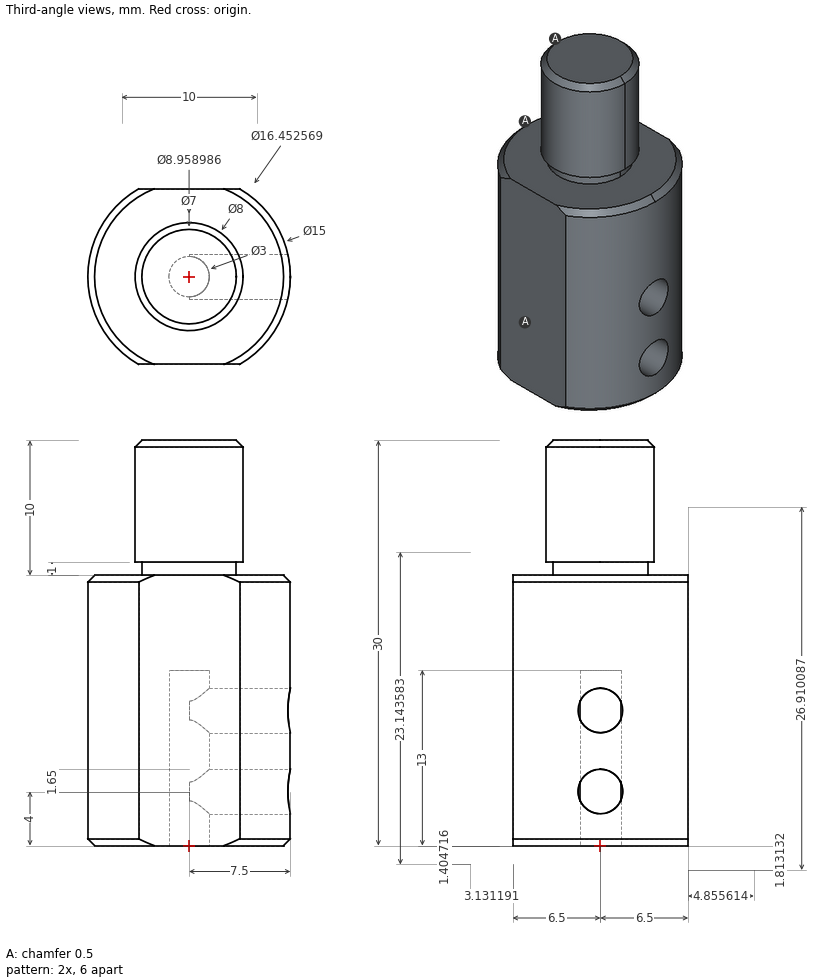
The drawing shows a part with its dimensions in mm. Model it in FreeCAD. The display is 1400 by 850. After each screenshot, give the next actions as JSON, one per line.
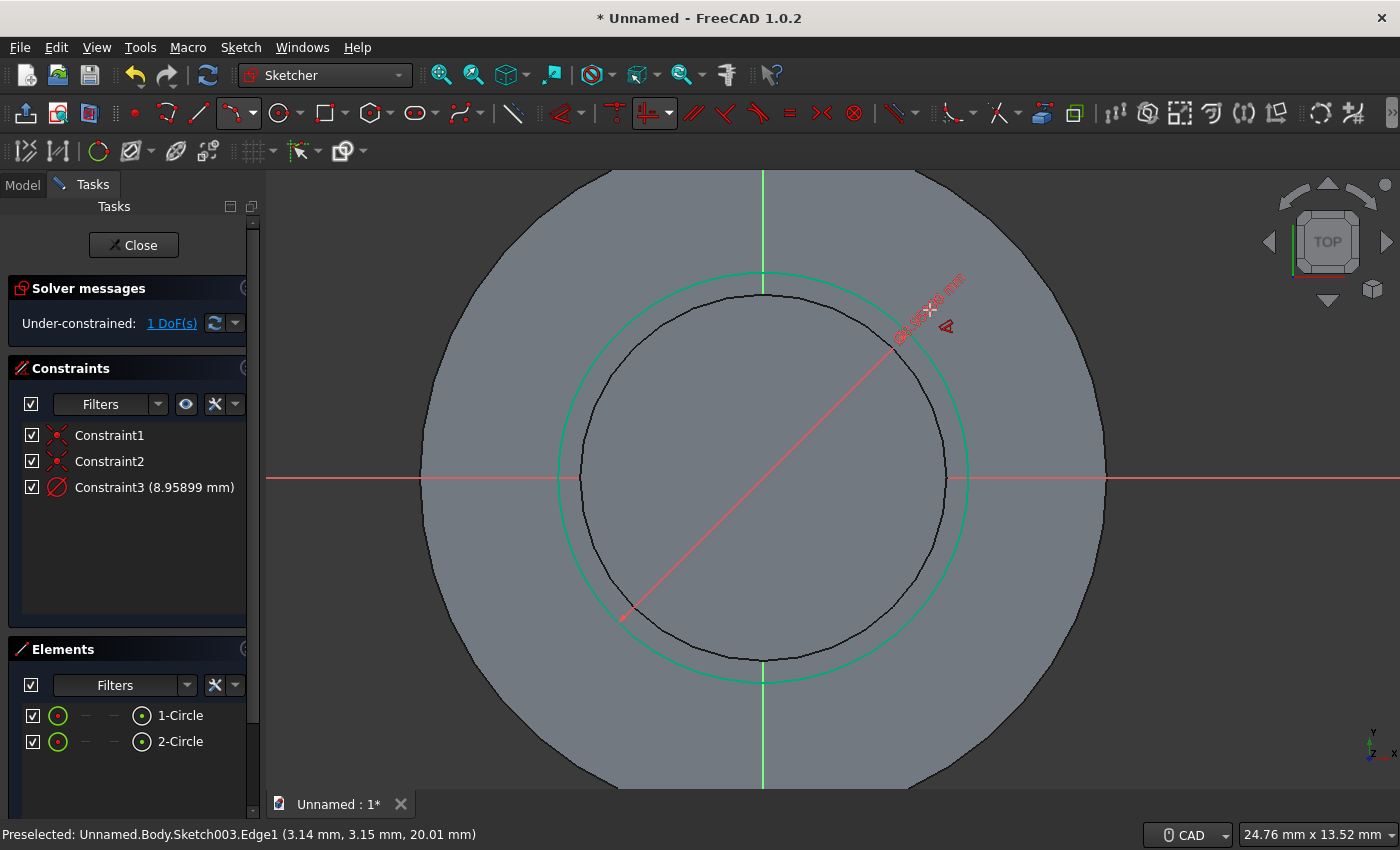
{"action": "left_click", "coordinate": [876, 364]}
{"action": "left_click", "coordinate": [899, 341]}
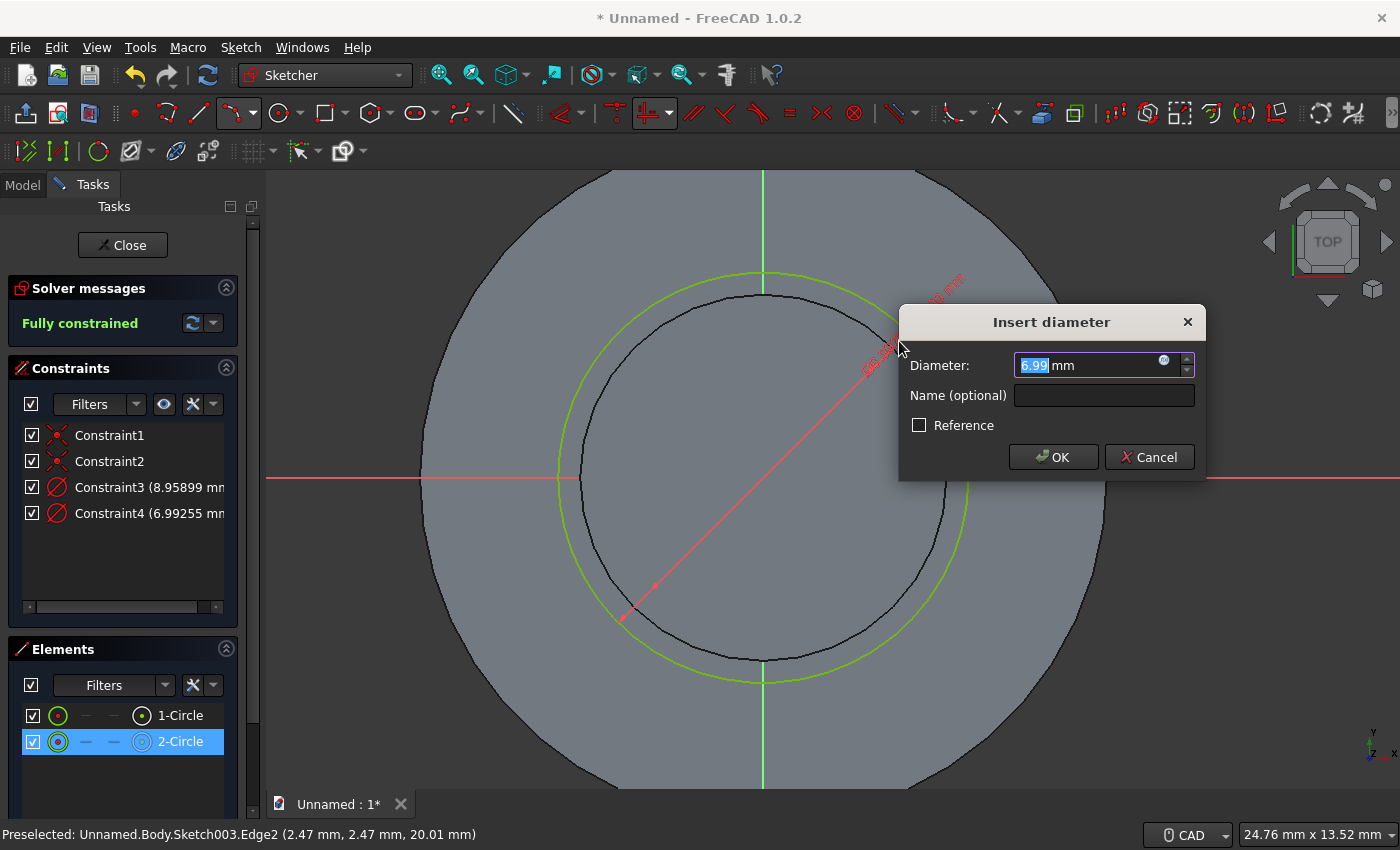
{"action": "type", "text": "7"}
{"action": "key", "text": "Return"}
{"action": "key", "text": "Escape"}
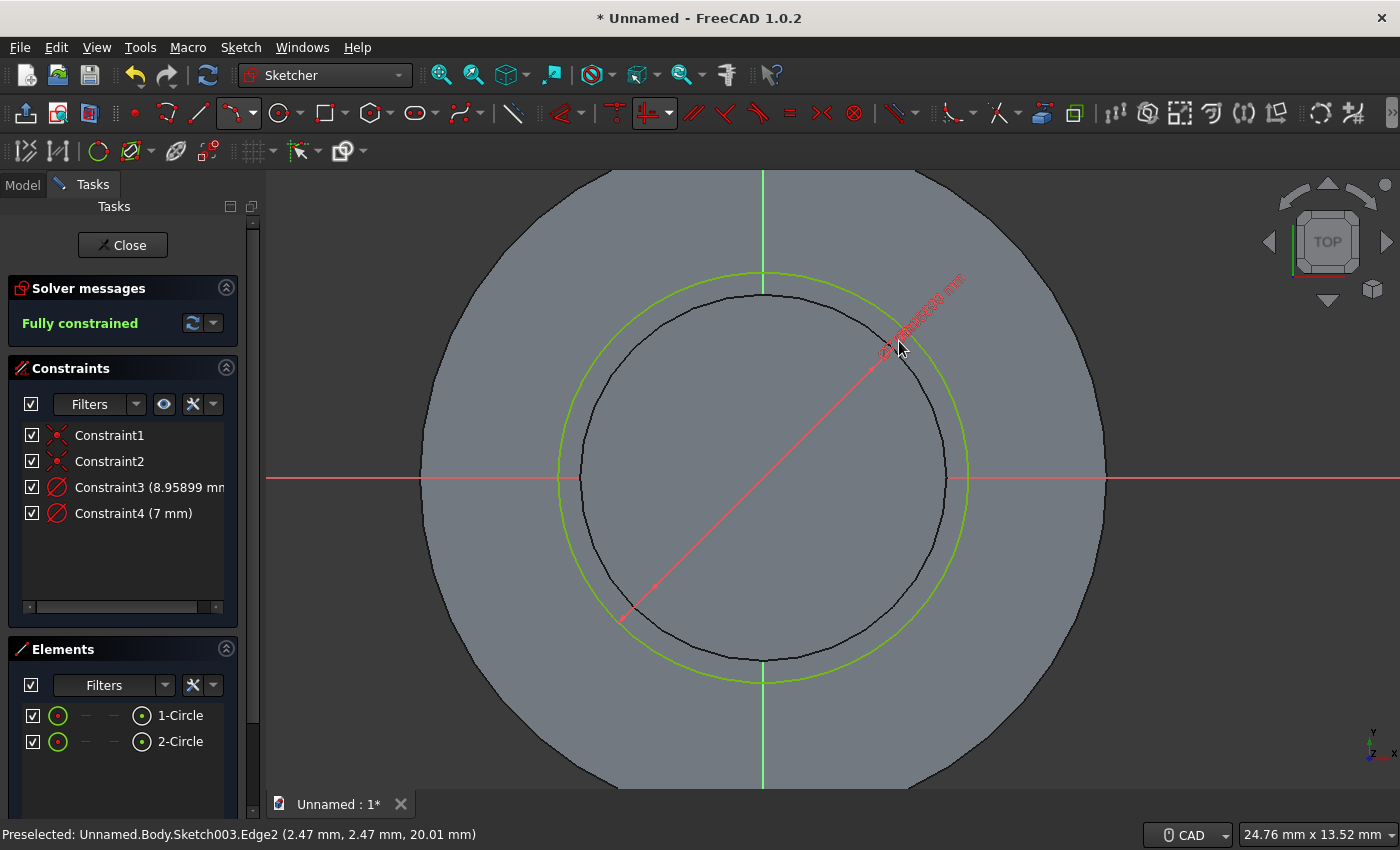
{"action": "left_click", "coordinate": [123, 245]}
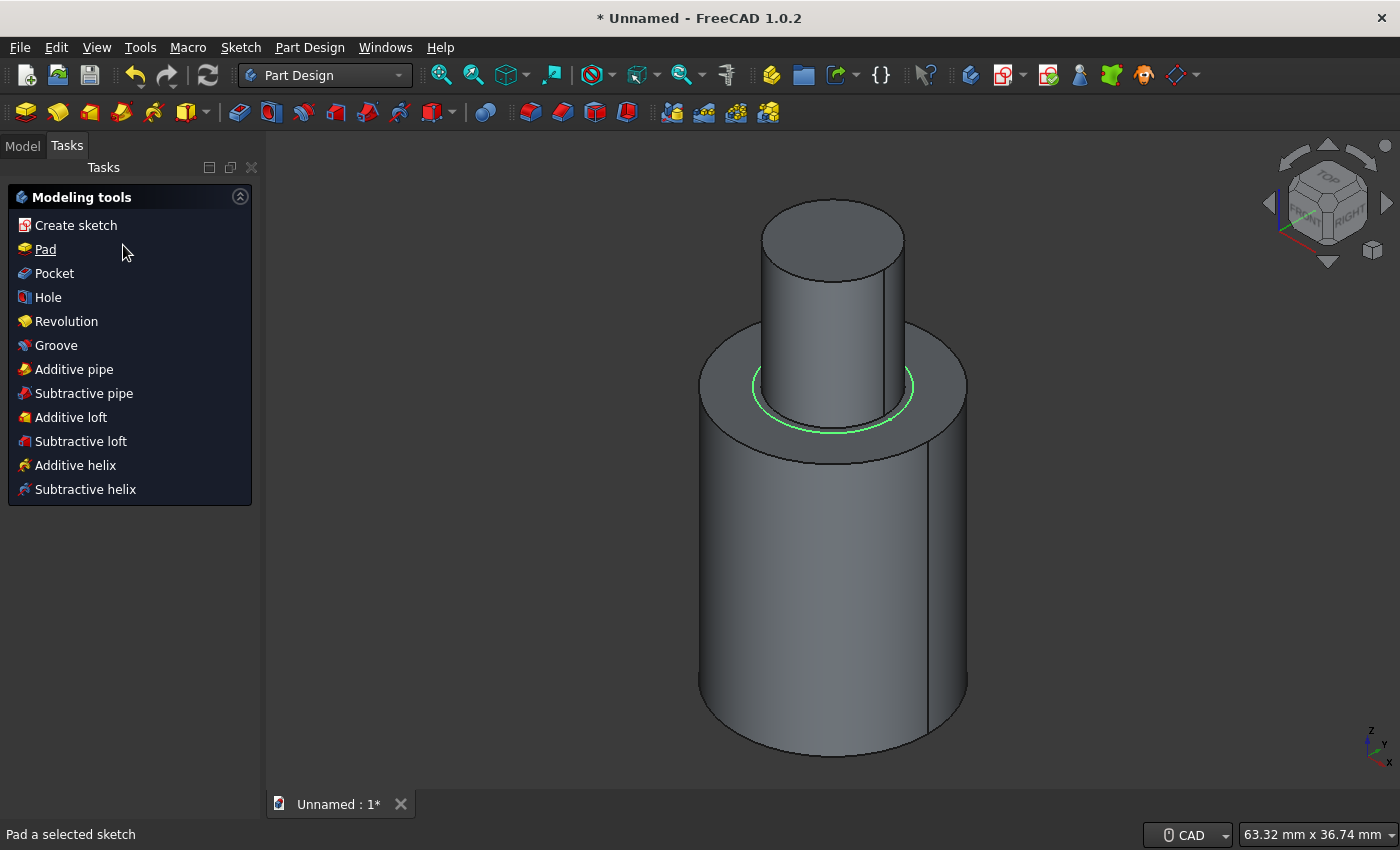
{"action": "left_click", "coordinate": [240, 112]}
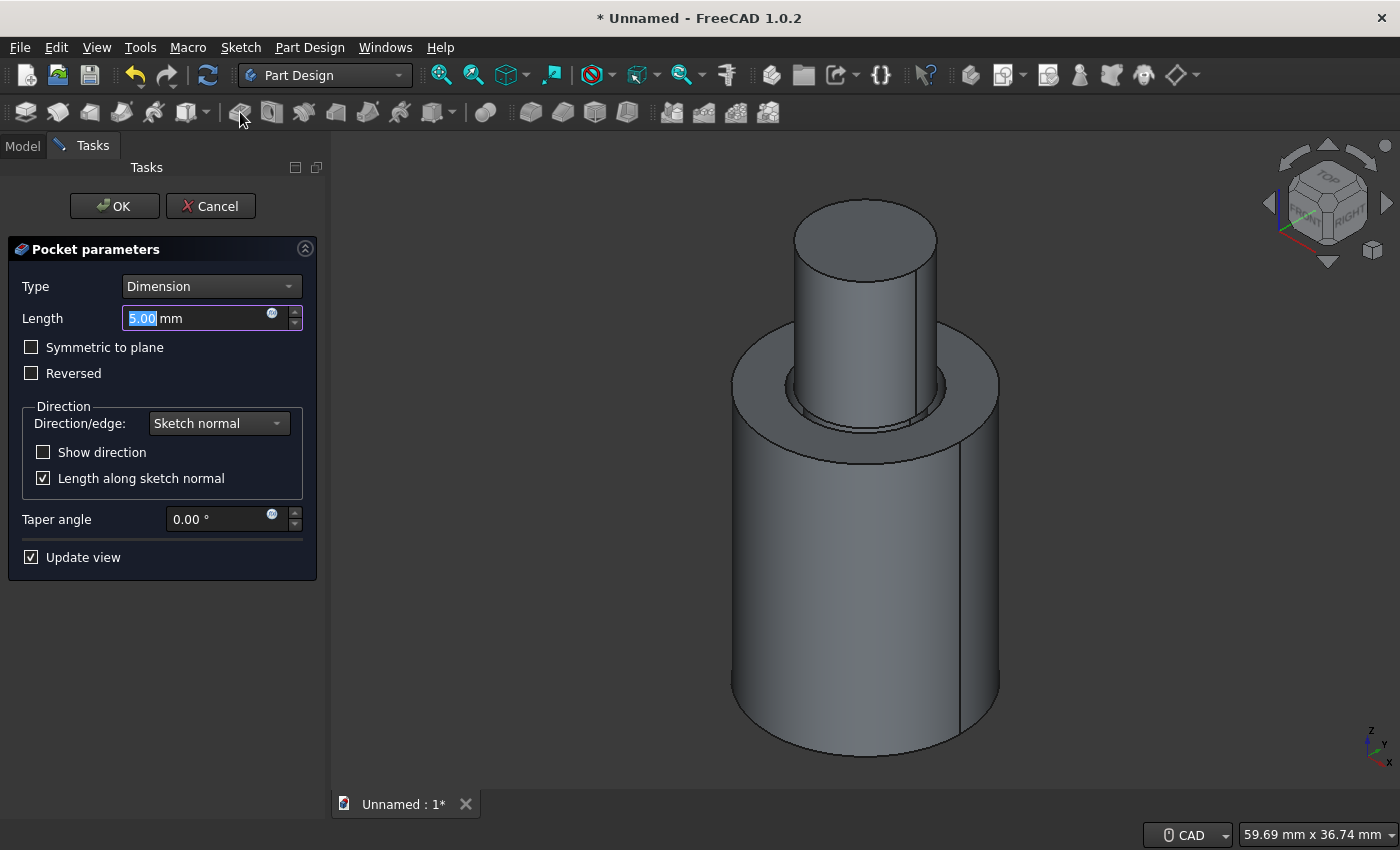
{"action": "type", "text": "1"}
{"action": "key", "text": "Tab"}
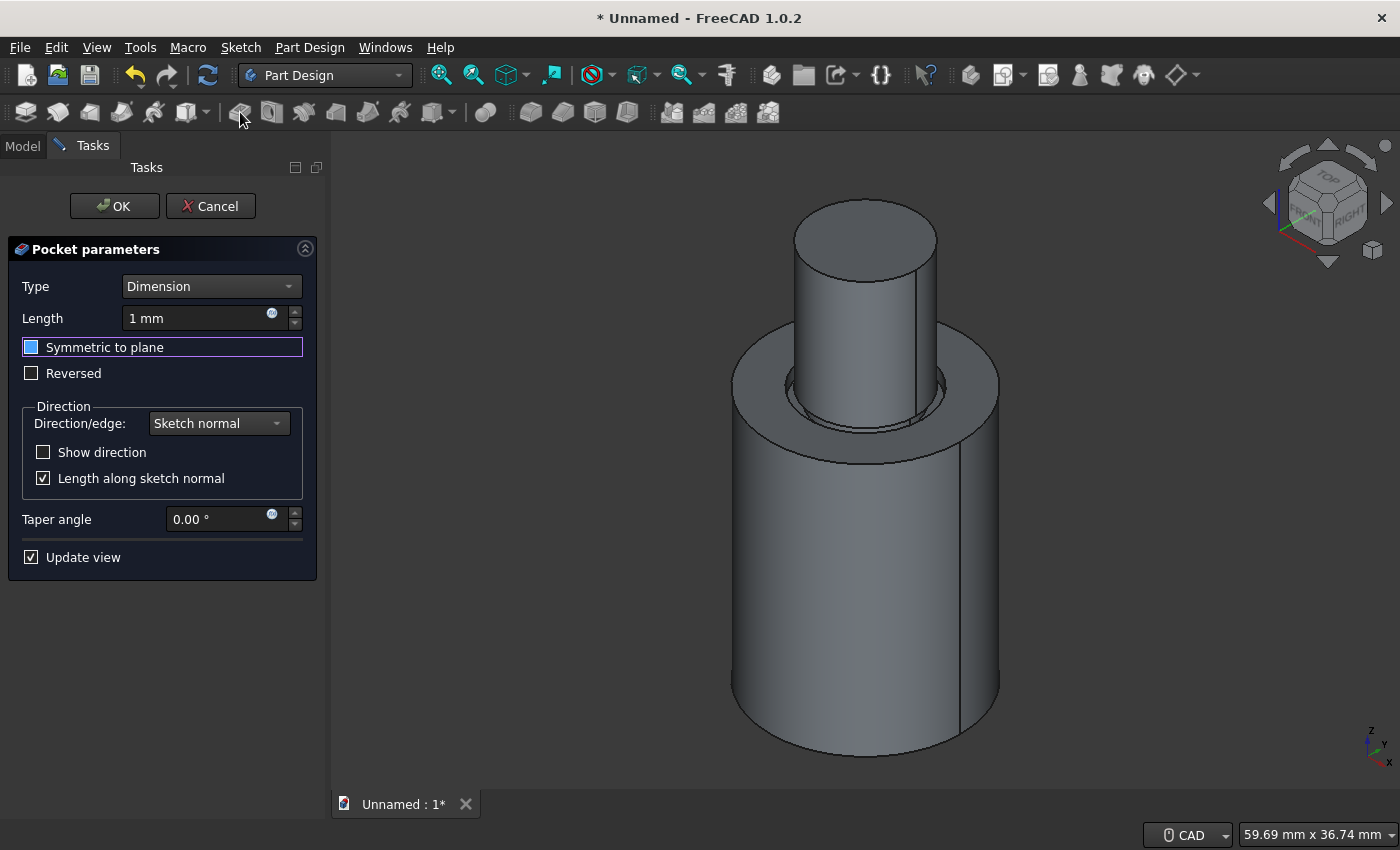
{"action": "left_click", "coordinate": [30, 373]}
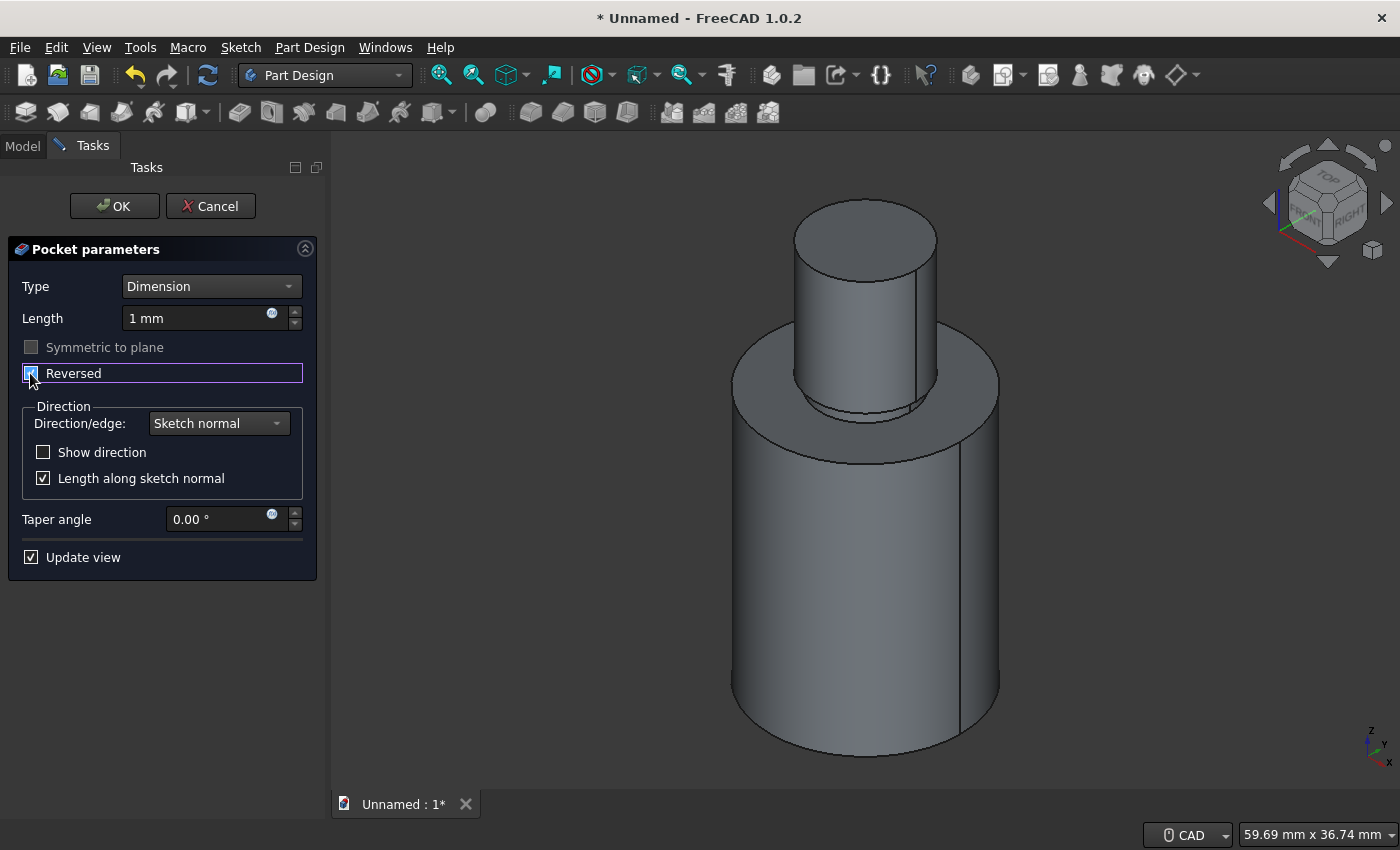
{"action": "left_click", "coordinate": [115, 206]}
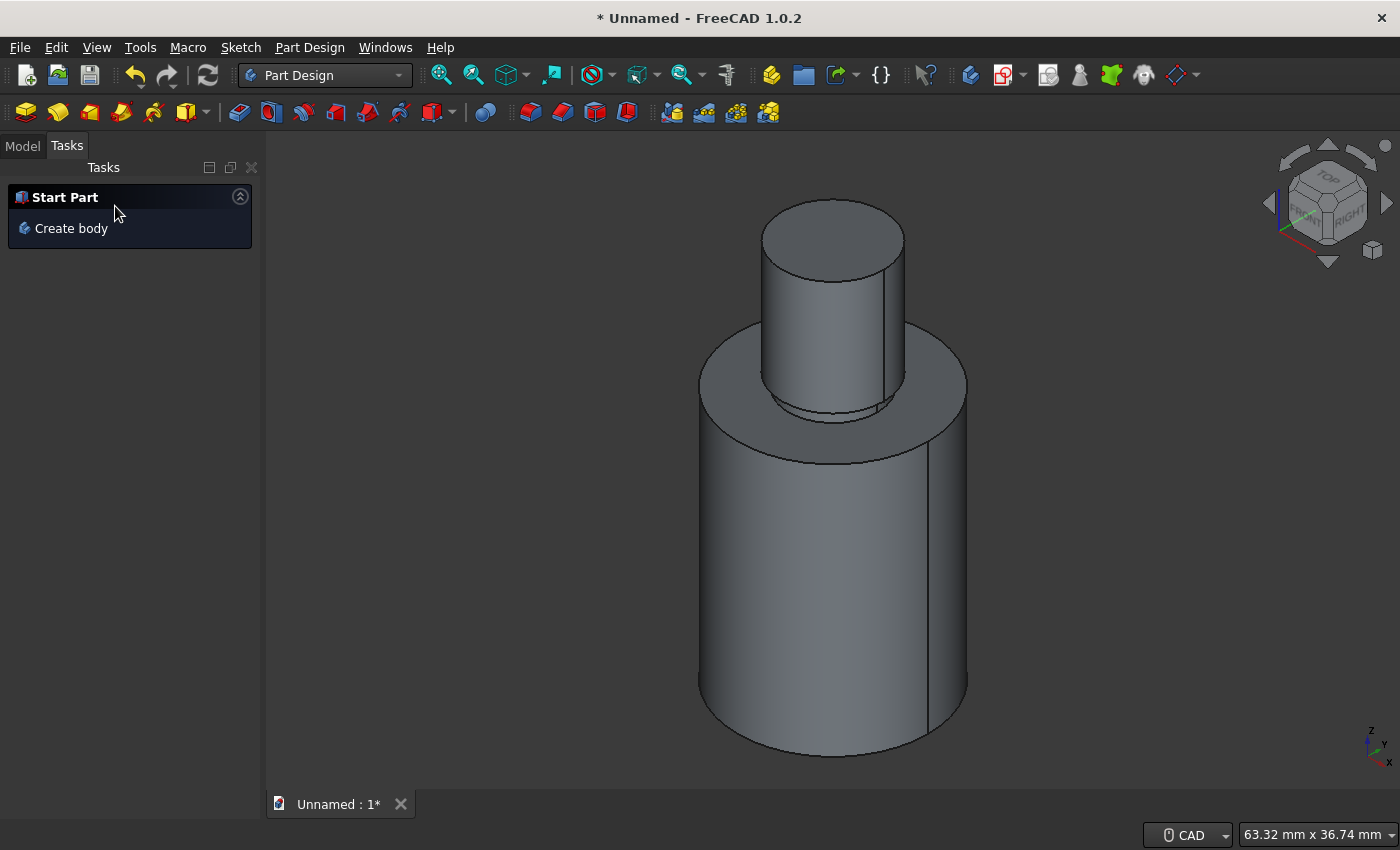
{"action": "left_click", "coordinate": [442, 76]}